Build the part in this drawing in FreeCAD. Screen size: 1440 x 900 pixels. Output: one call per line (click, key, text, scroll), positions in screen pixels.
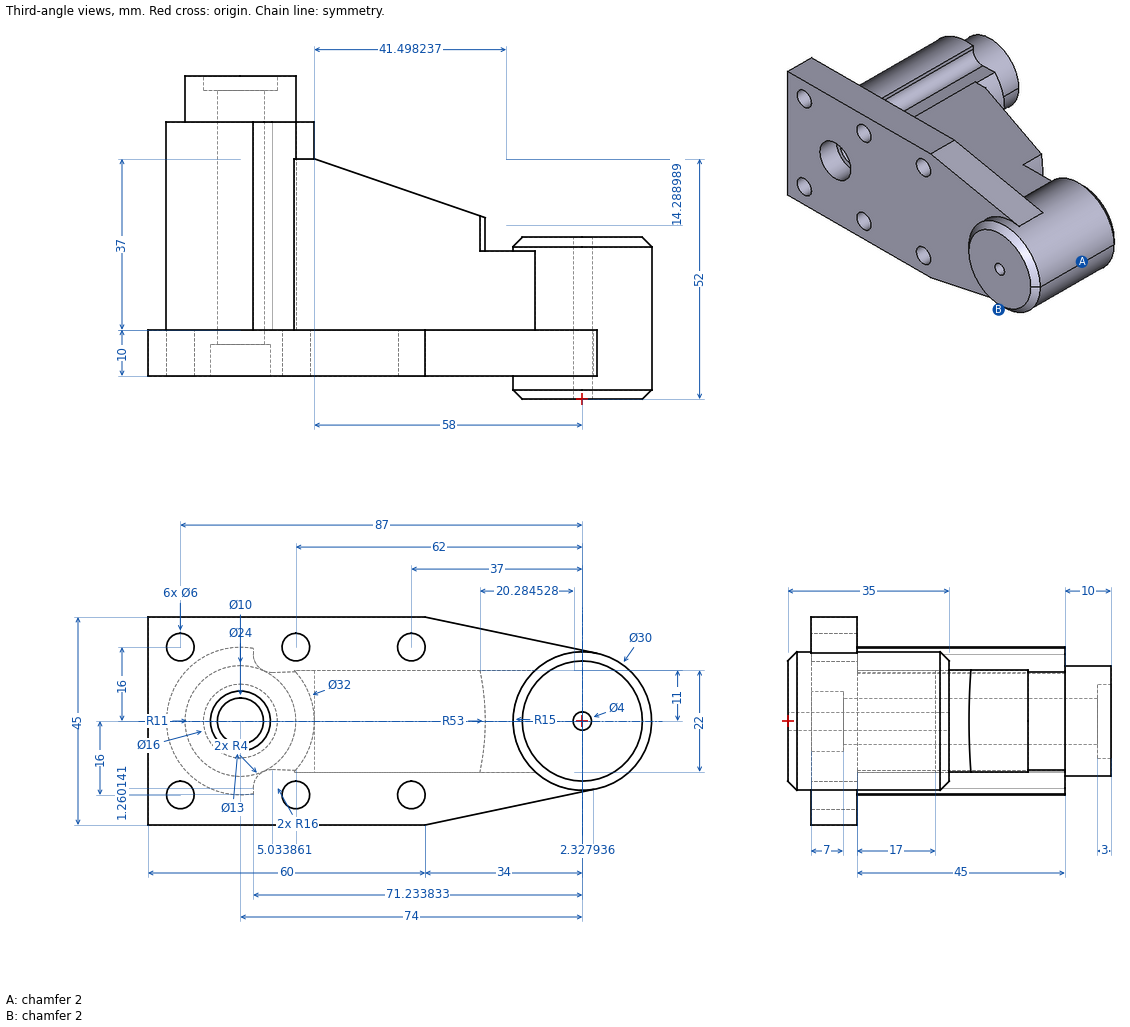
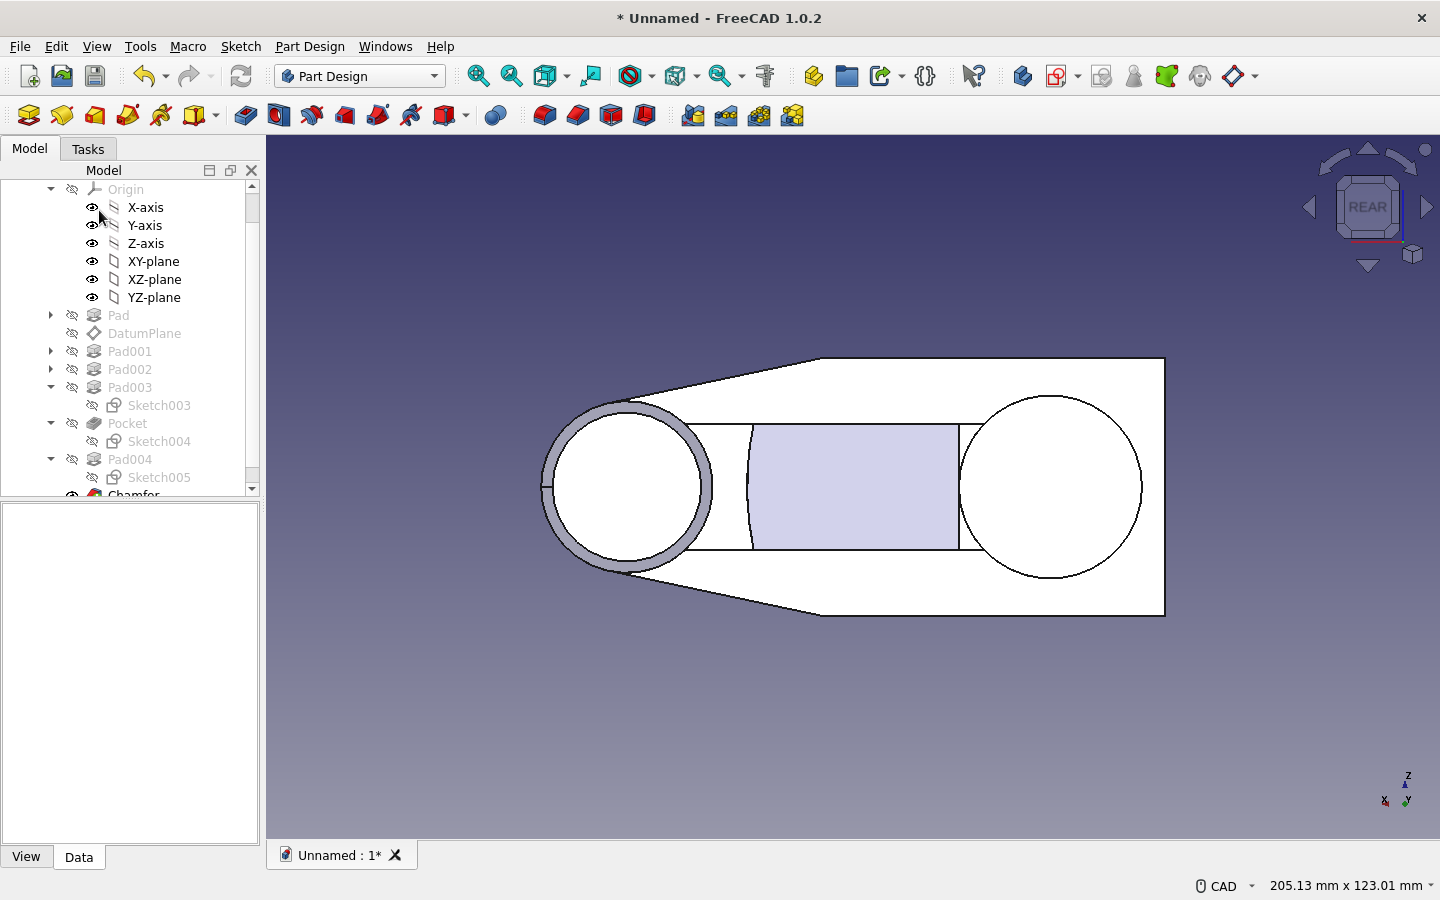
key(0)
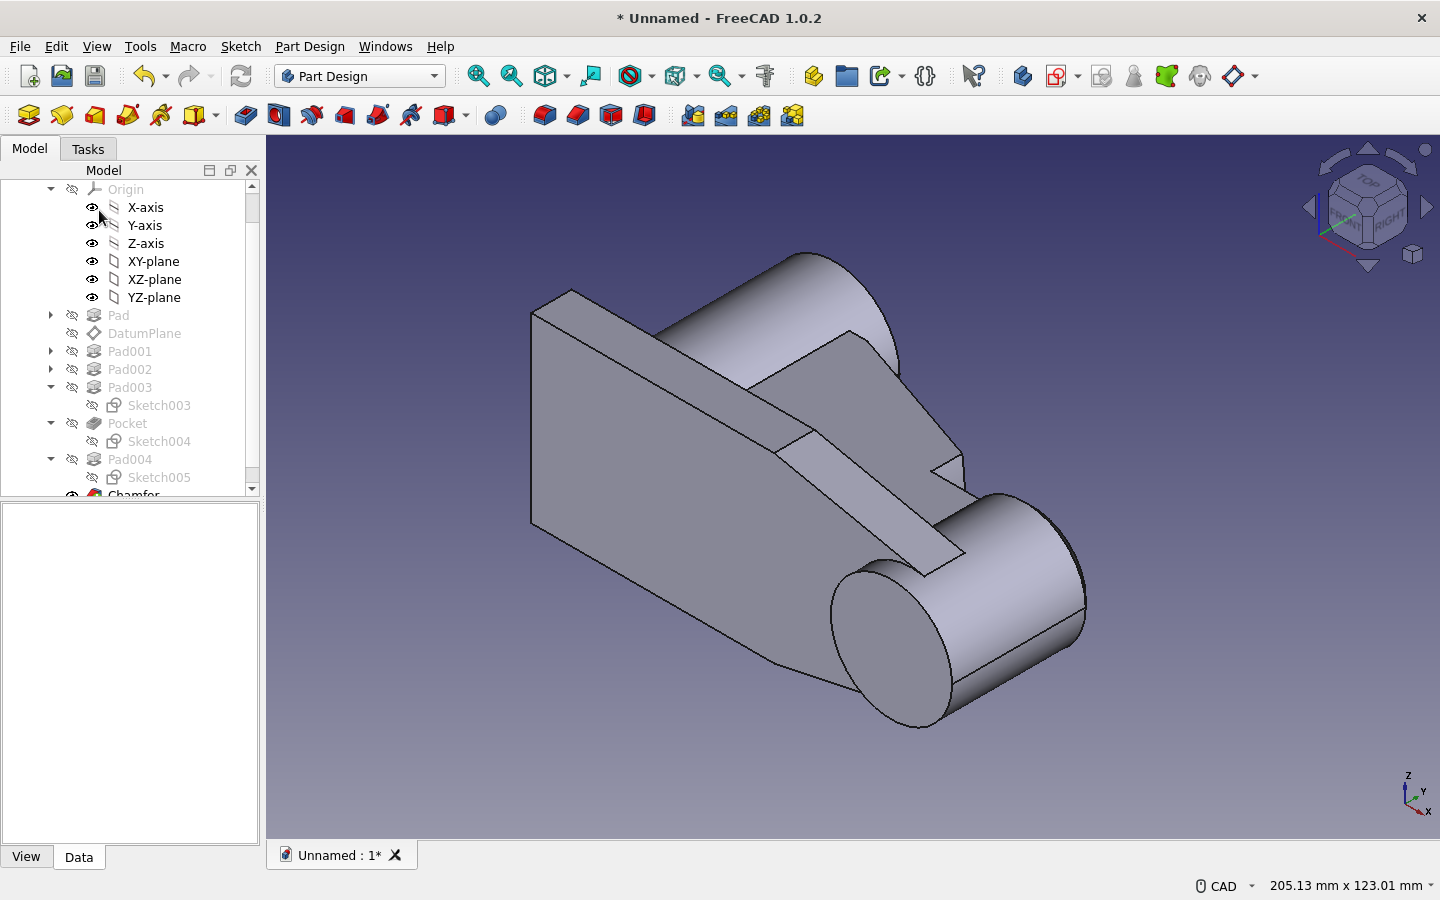
click(873, 571)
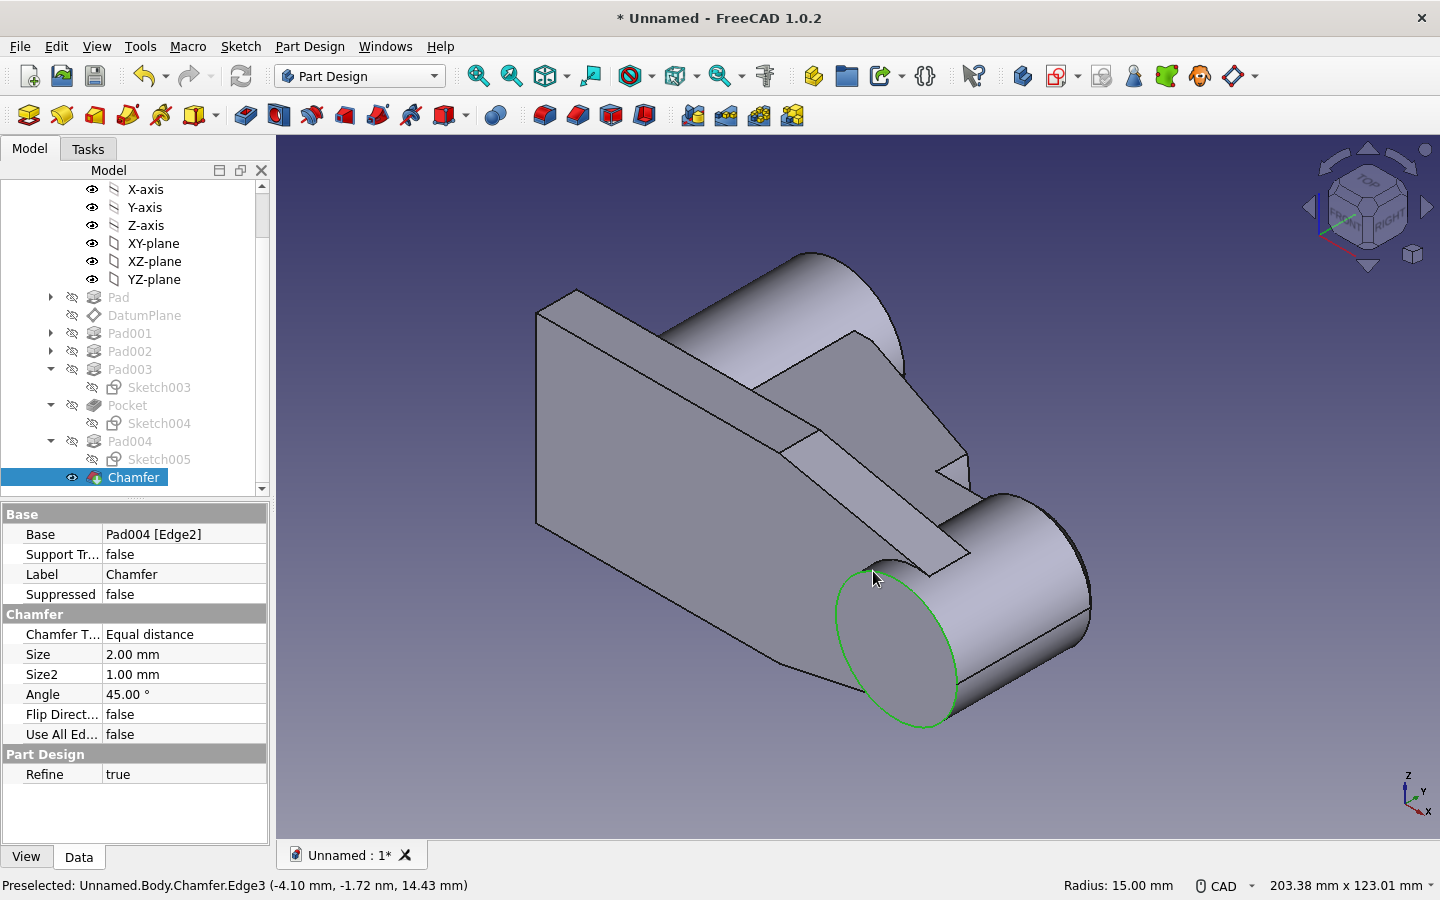
click(578, 116)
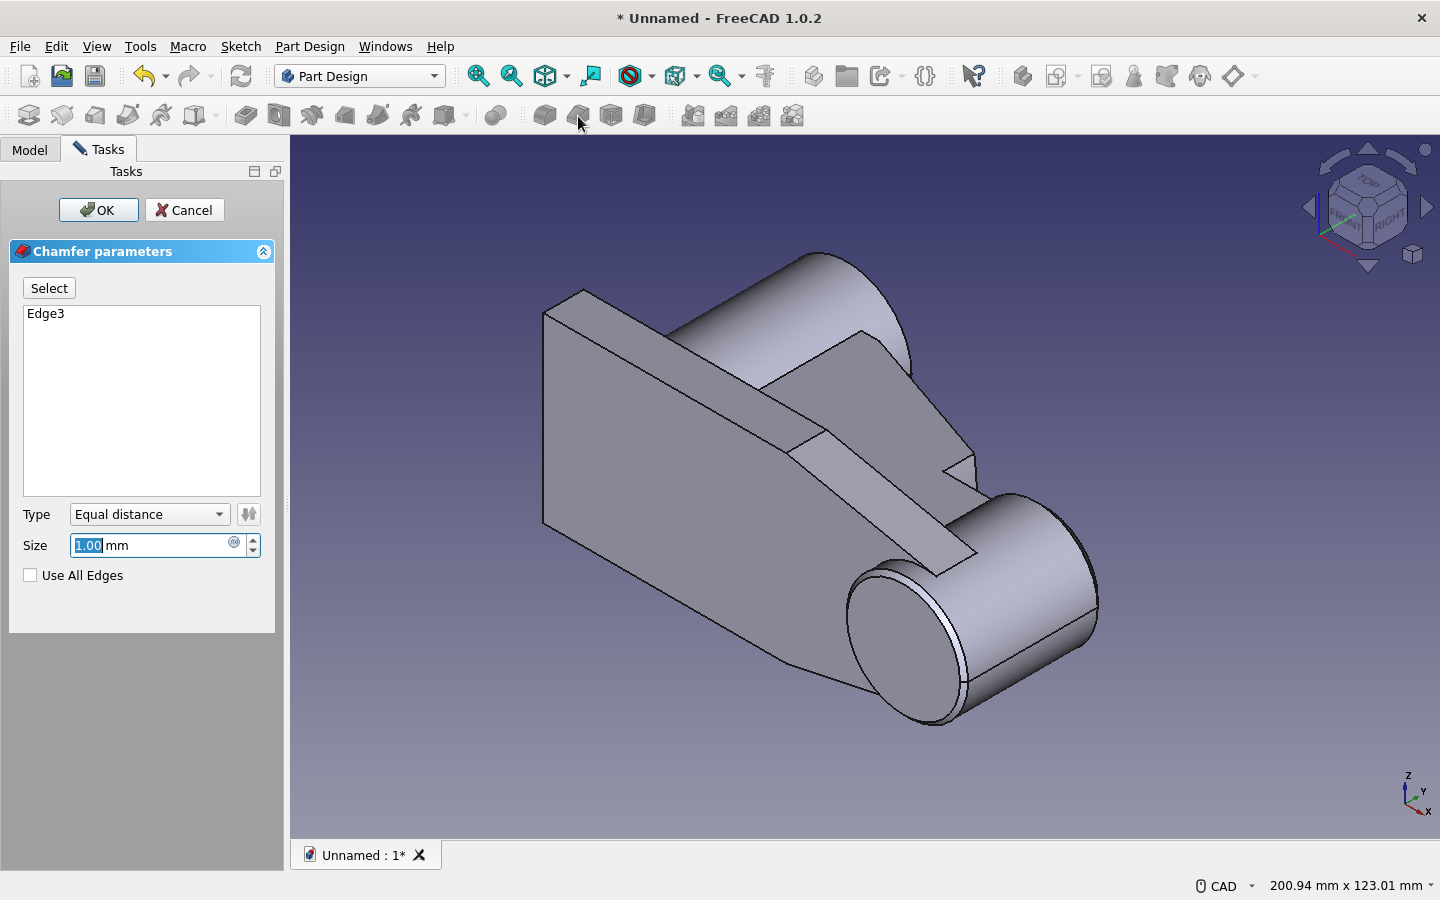
text(2)
key(Tab)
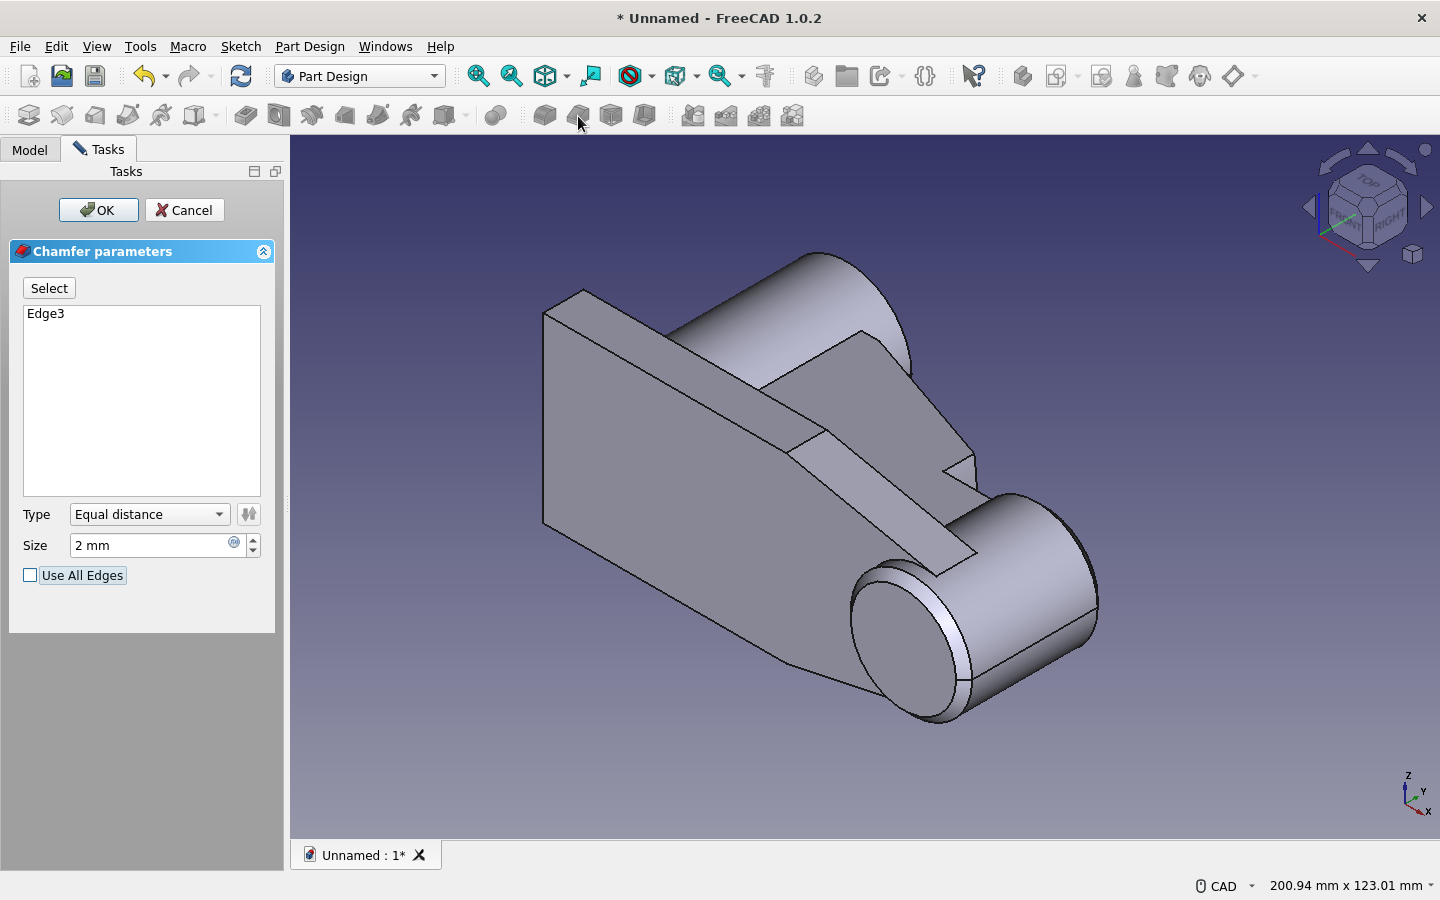
click(99, 210)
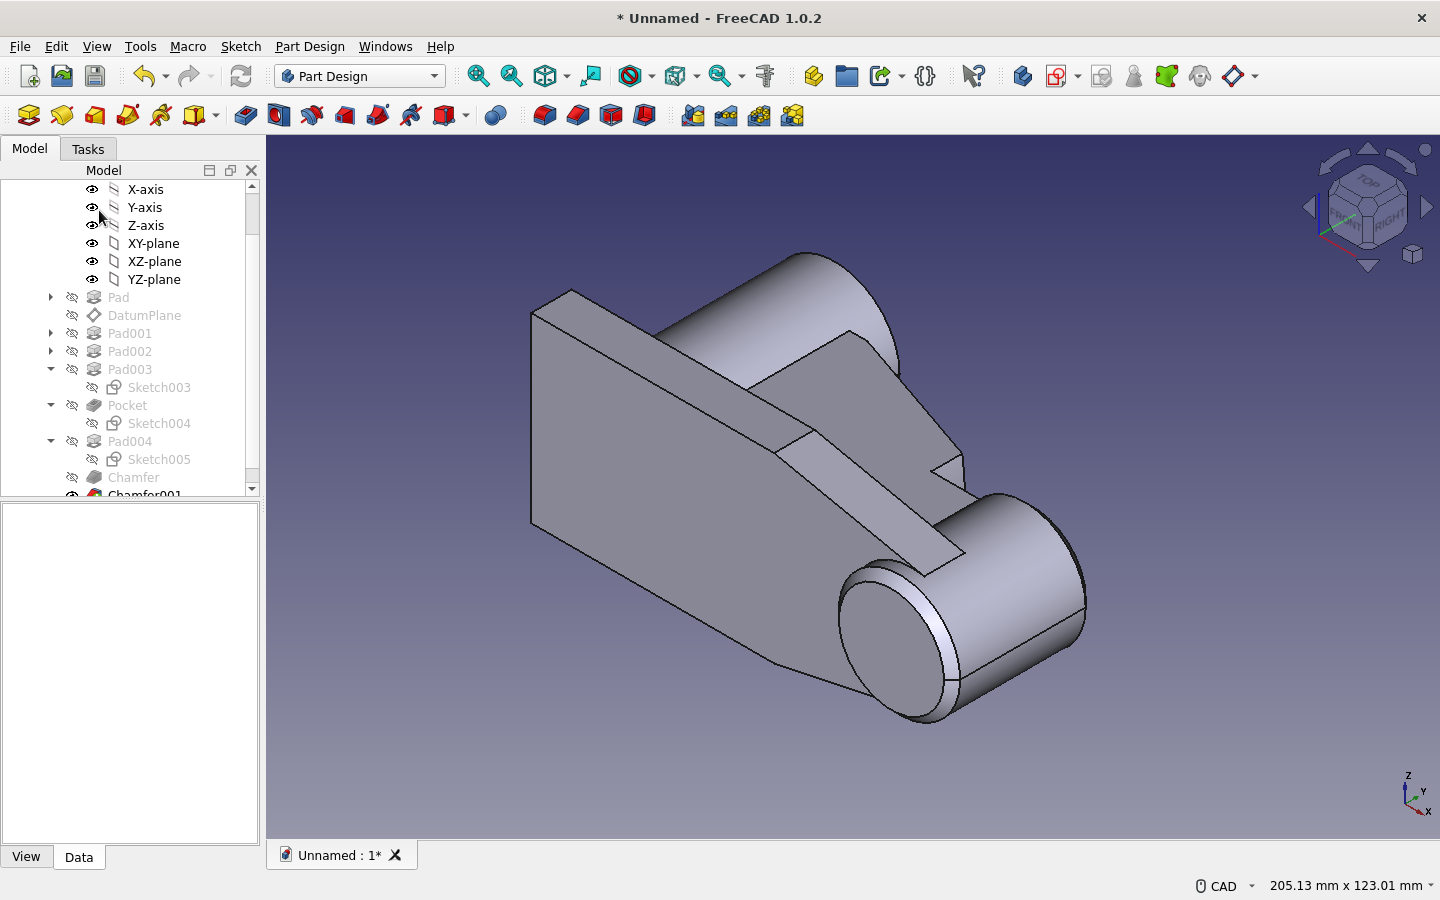
key(4)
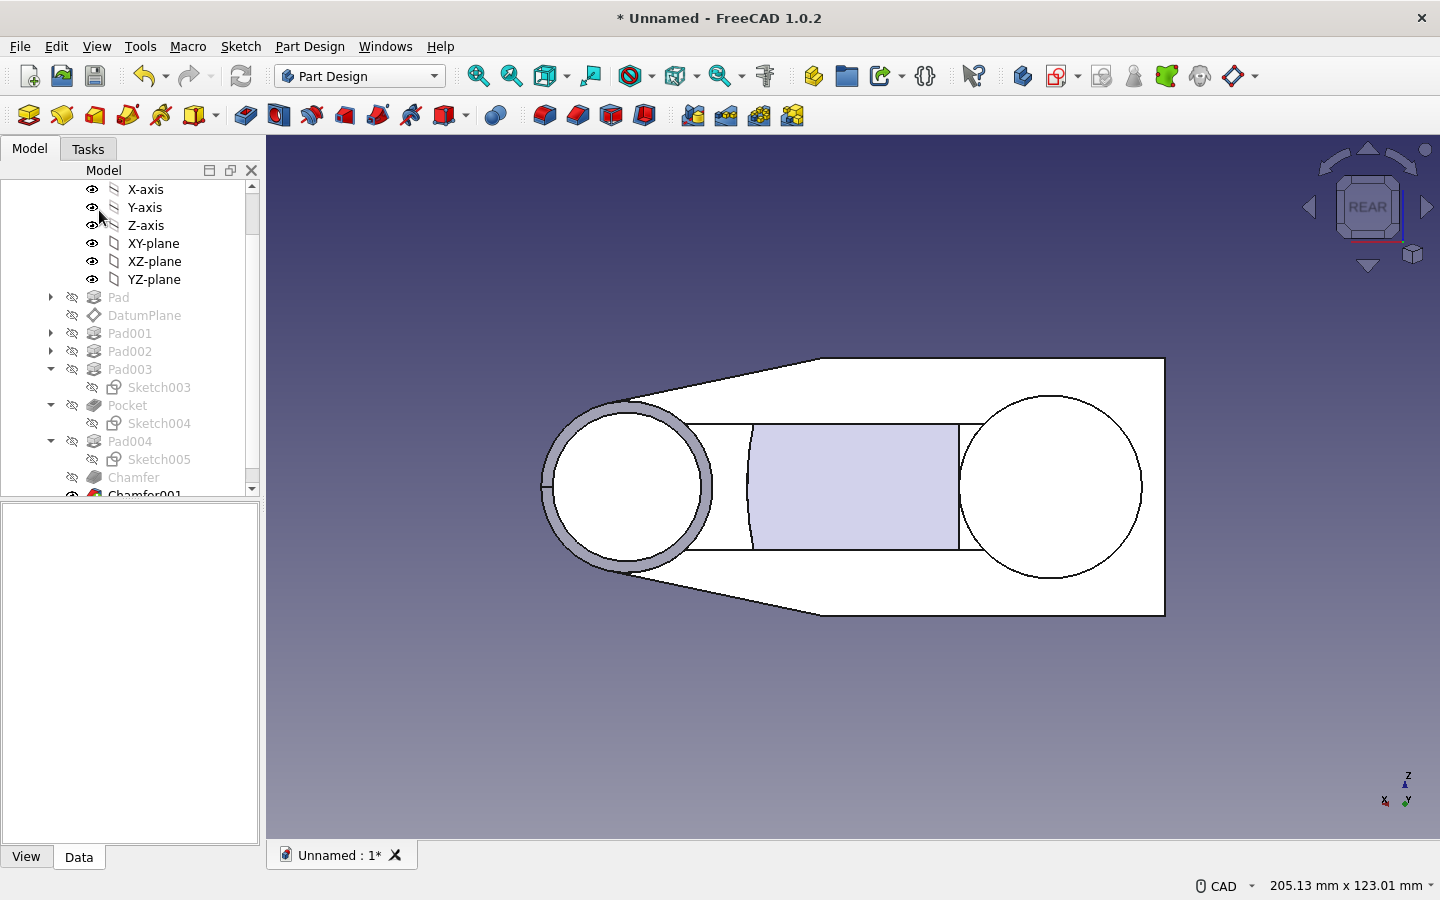
click(627, 486)